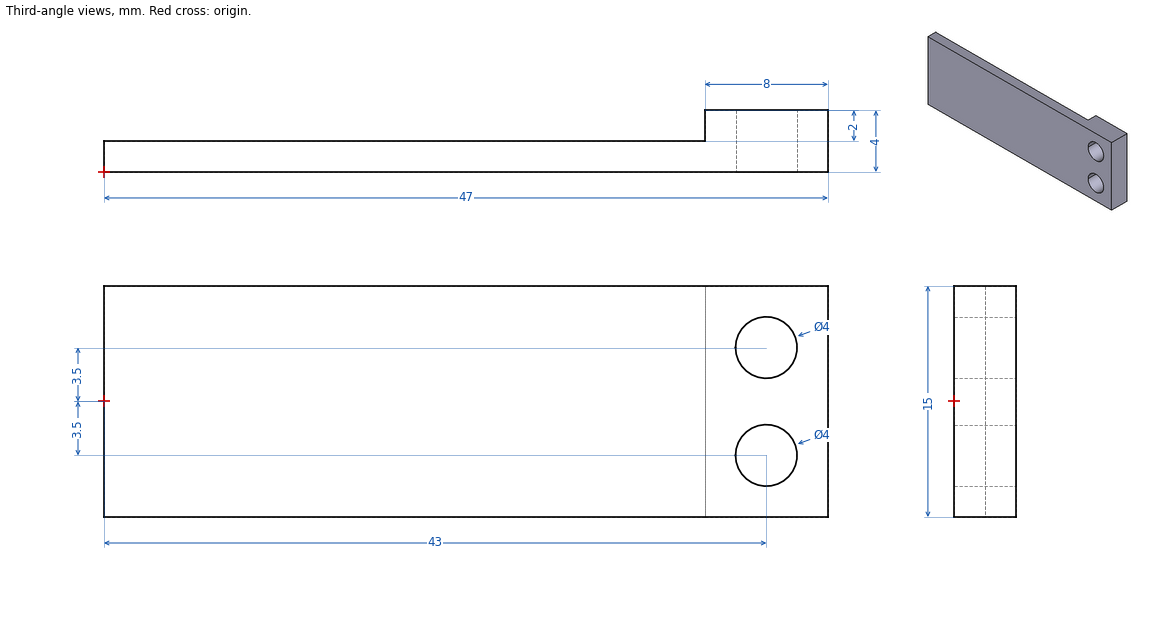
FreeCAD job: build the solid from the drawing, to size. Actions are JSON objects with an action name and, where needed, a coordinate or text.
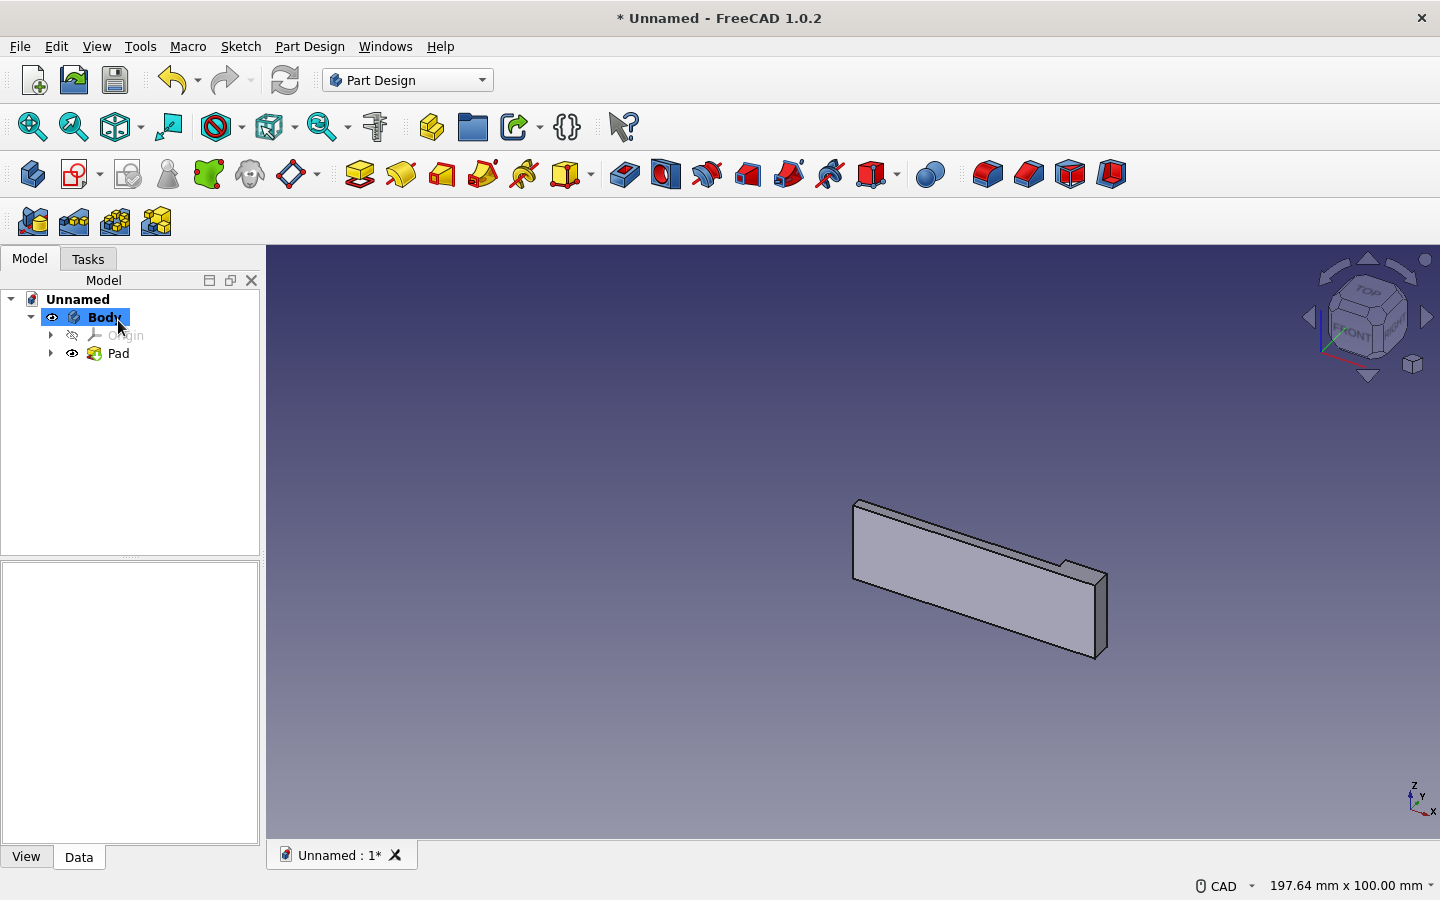
{"action": "left_click", "coordinate": [33, 128]}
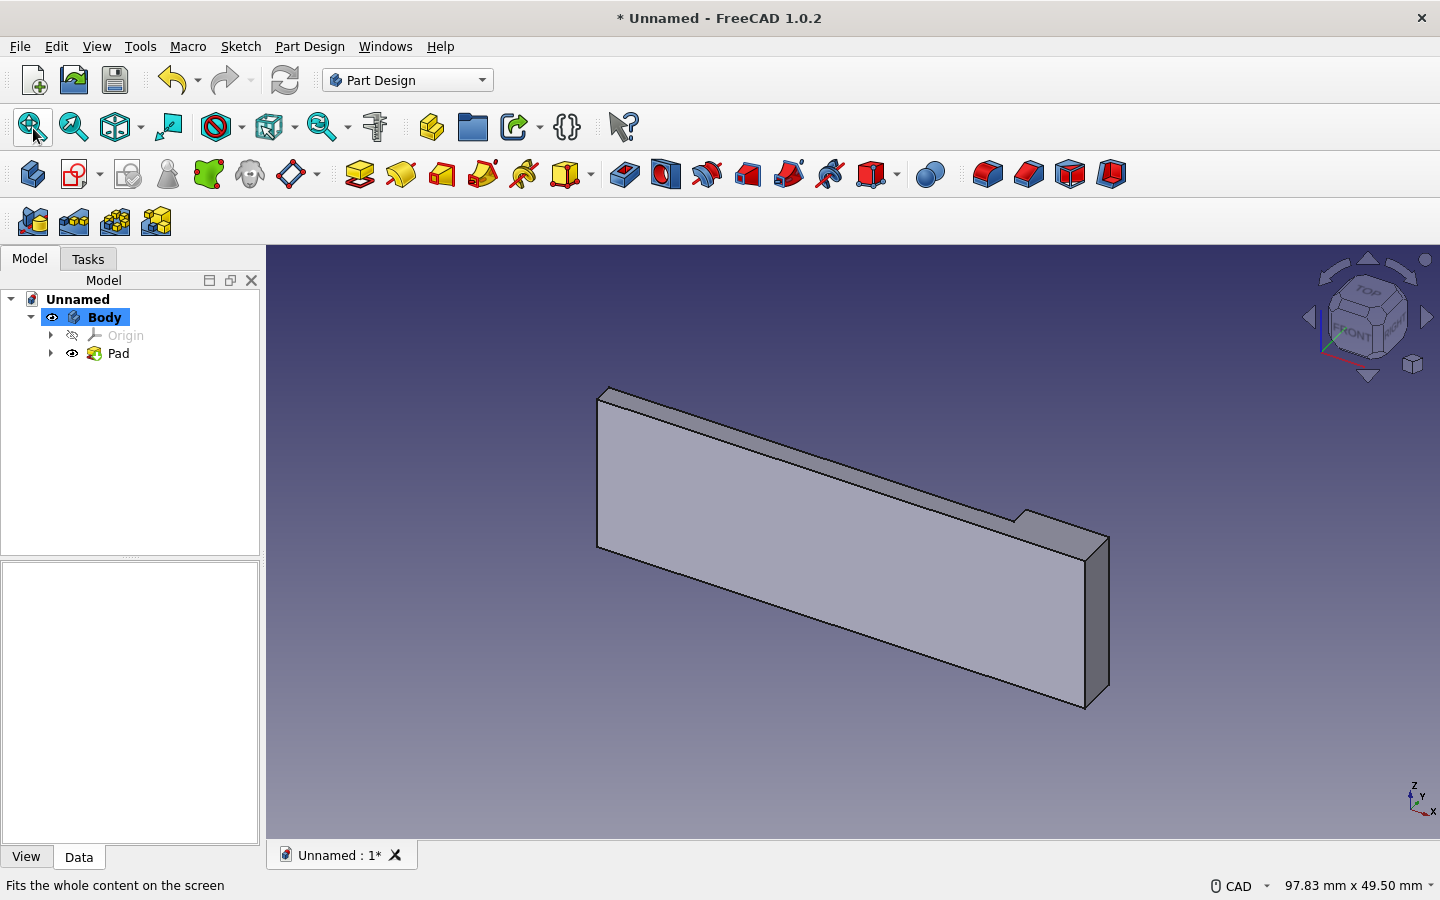
{"action": "key", "text": "4"}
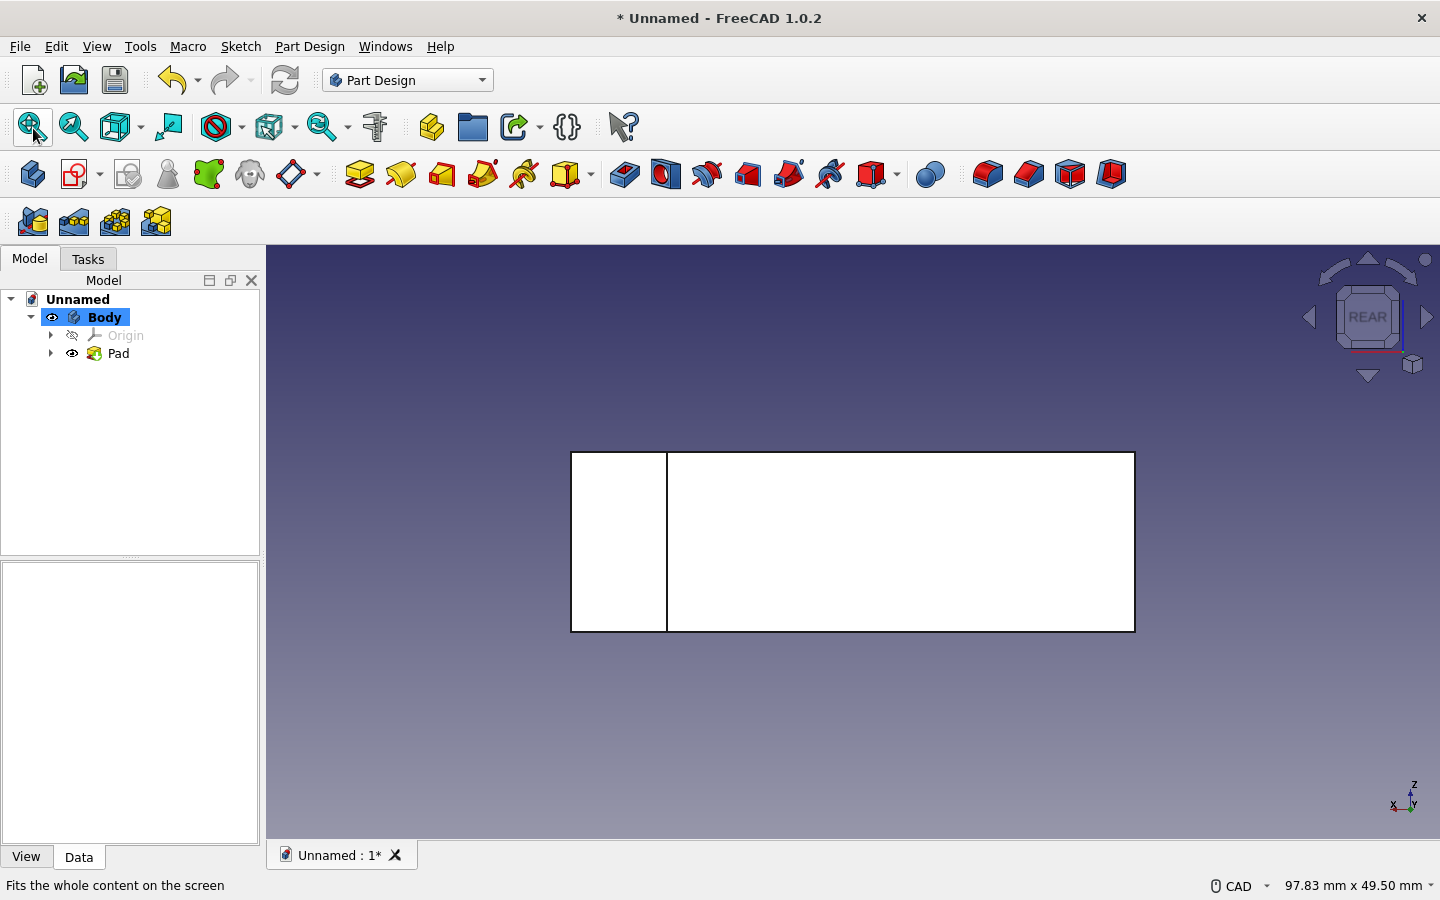
{"action": "left_click", "coordinate": [619, 515]}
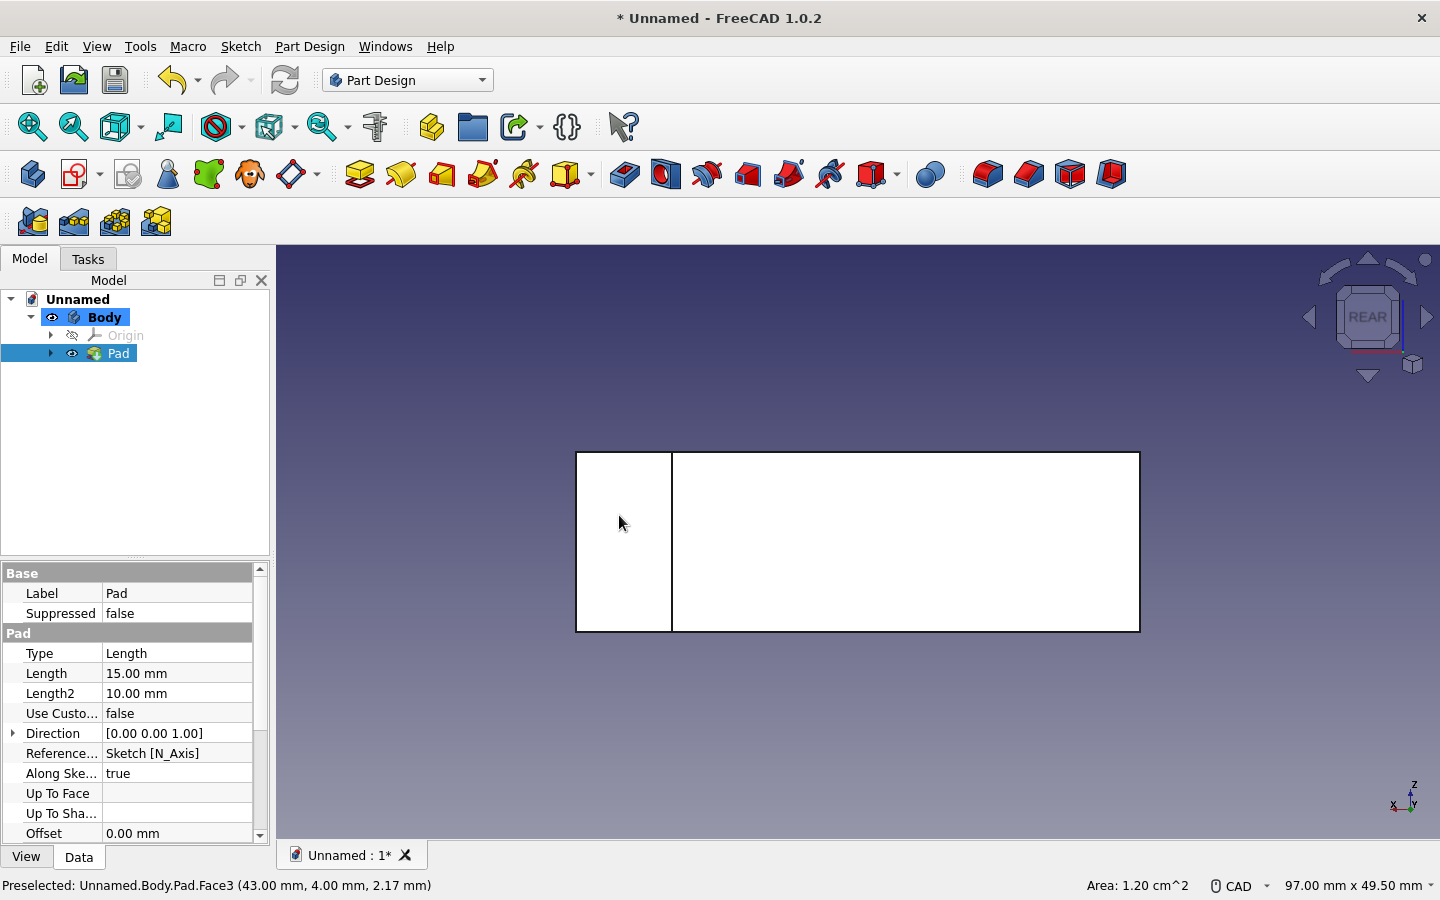
{"action": "left_click", "coordinate": [74, 174]}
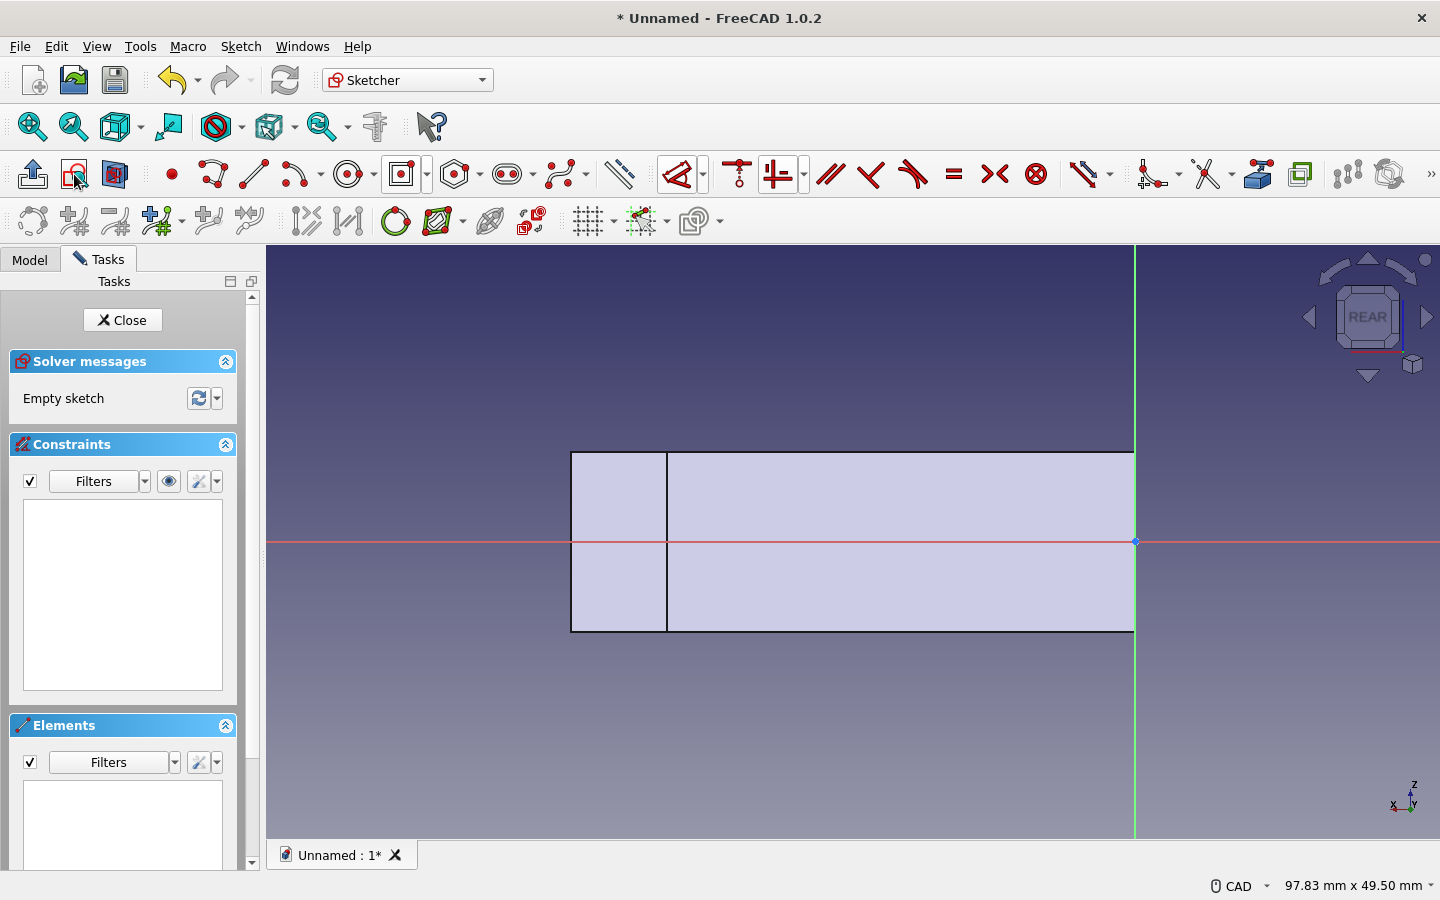
{"action": "scroll", "coordinate": [593, 591], "scroll_direction": "up", "scroll_amount": 10}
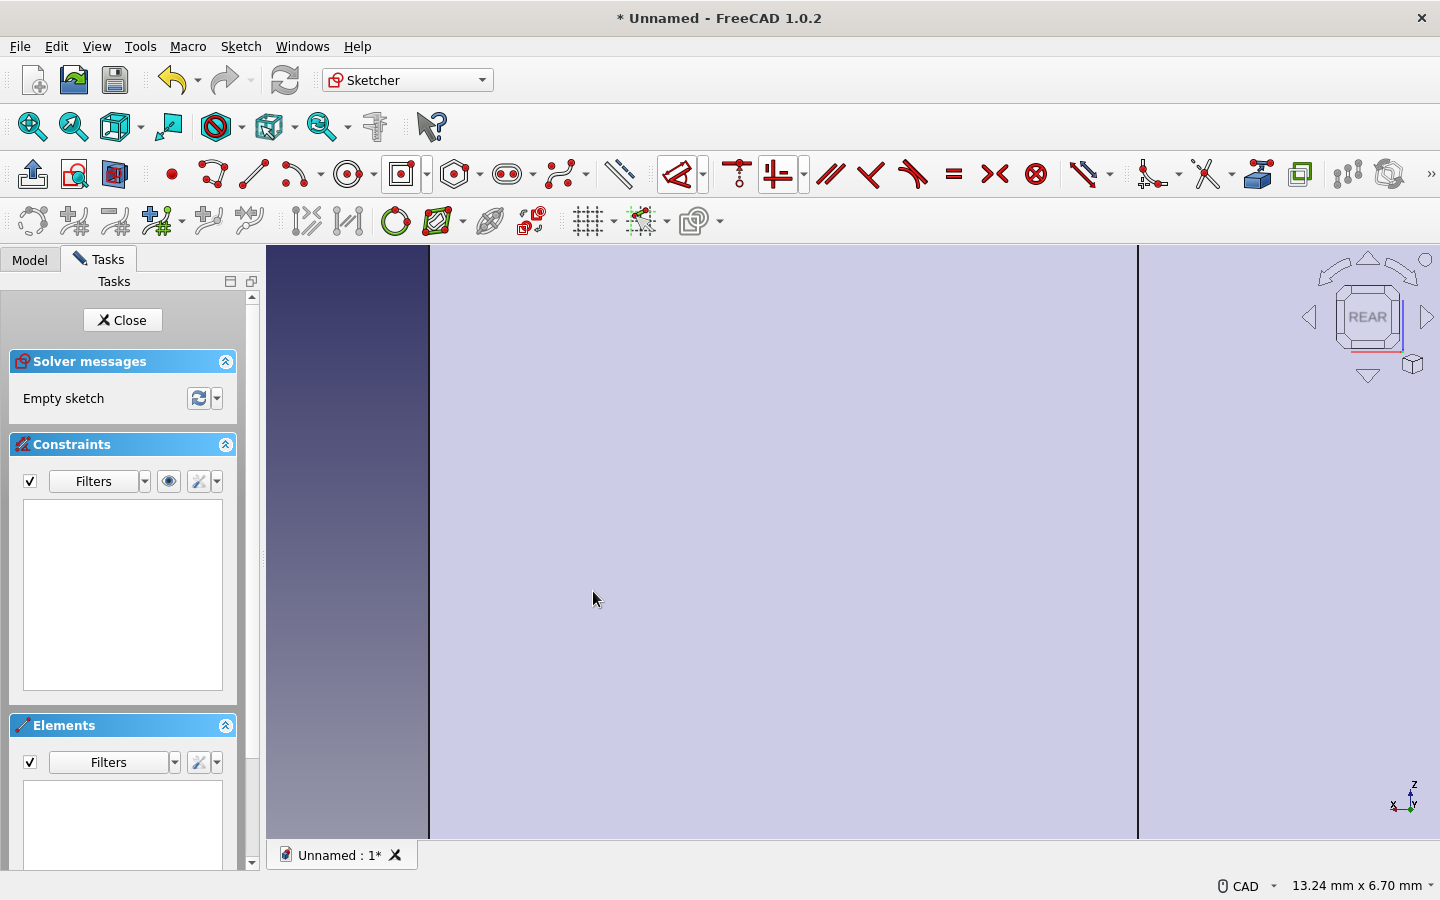
{"action": "left_click", "coordinate": [348, 174]}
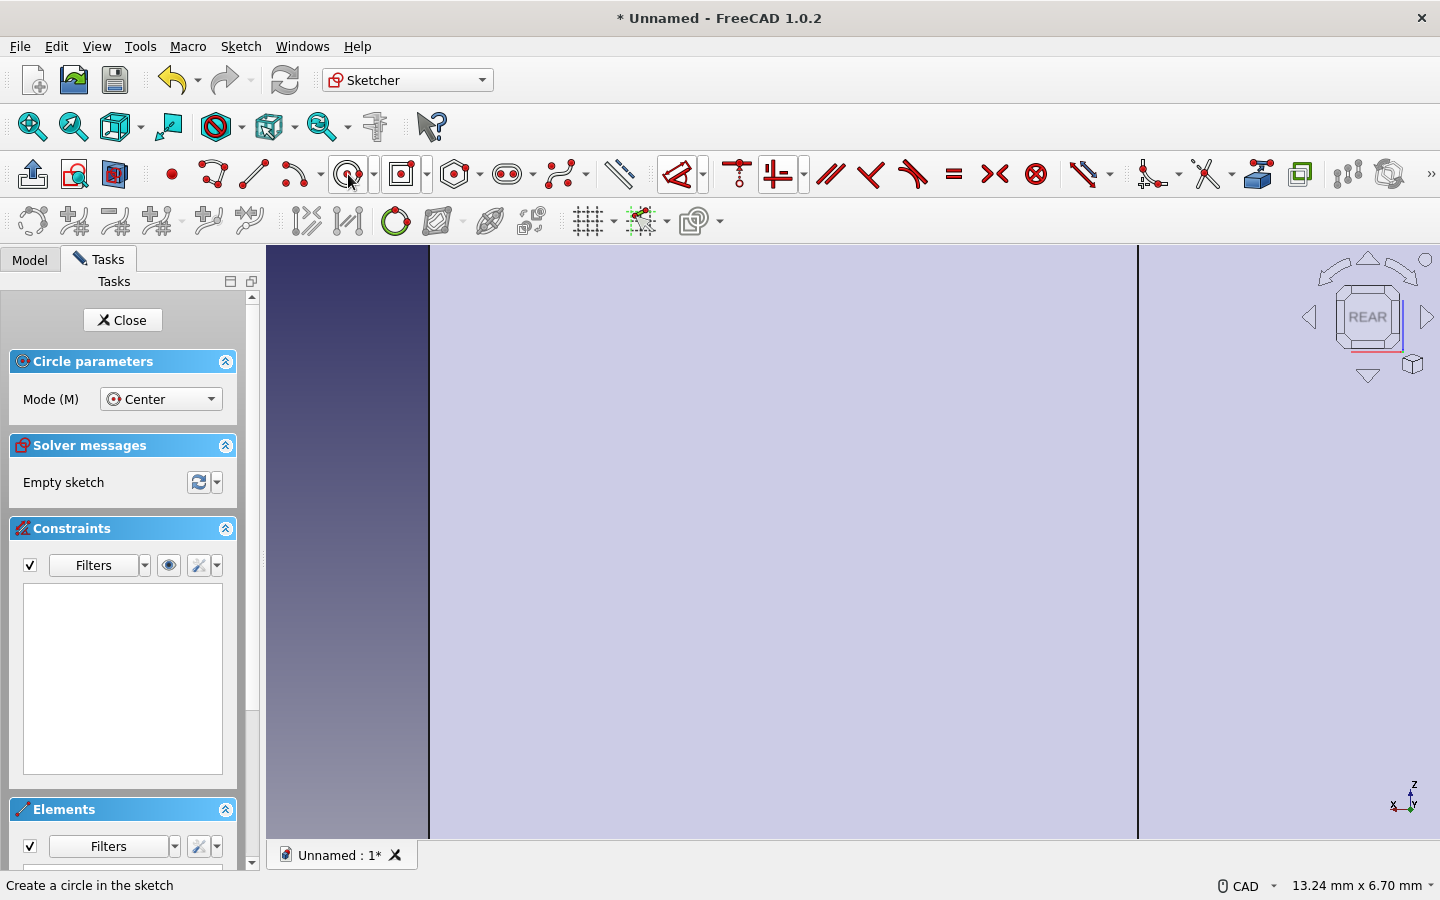
{"action": "left_click", "coordinate": [783, 536]}
{"action": "left_click", "coordinate": [909, 410]}
{"action": "key", "text": "Escape"}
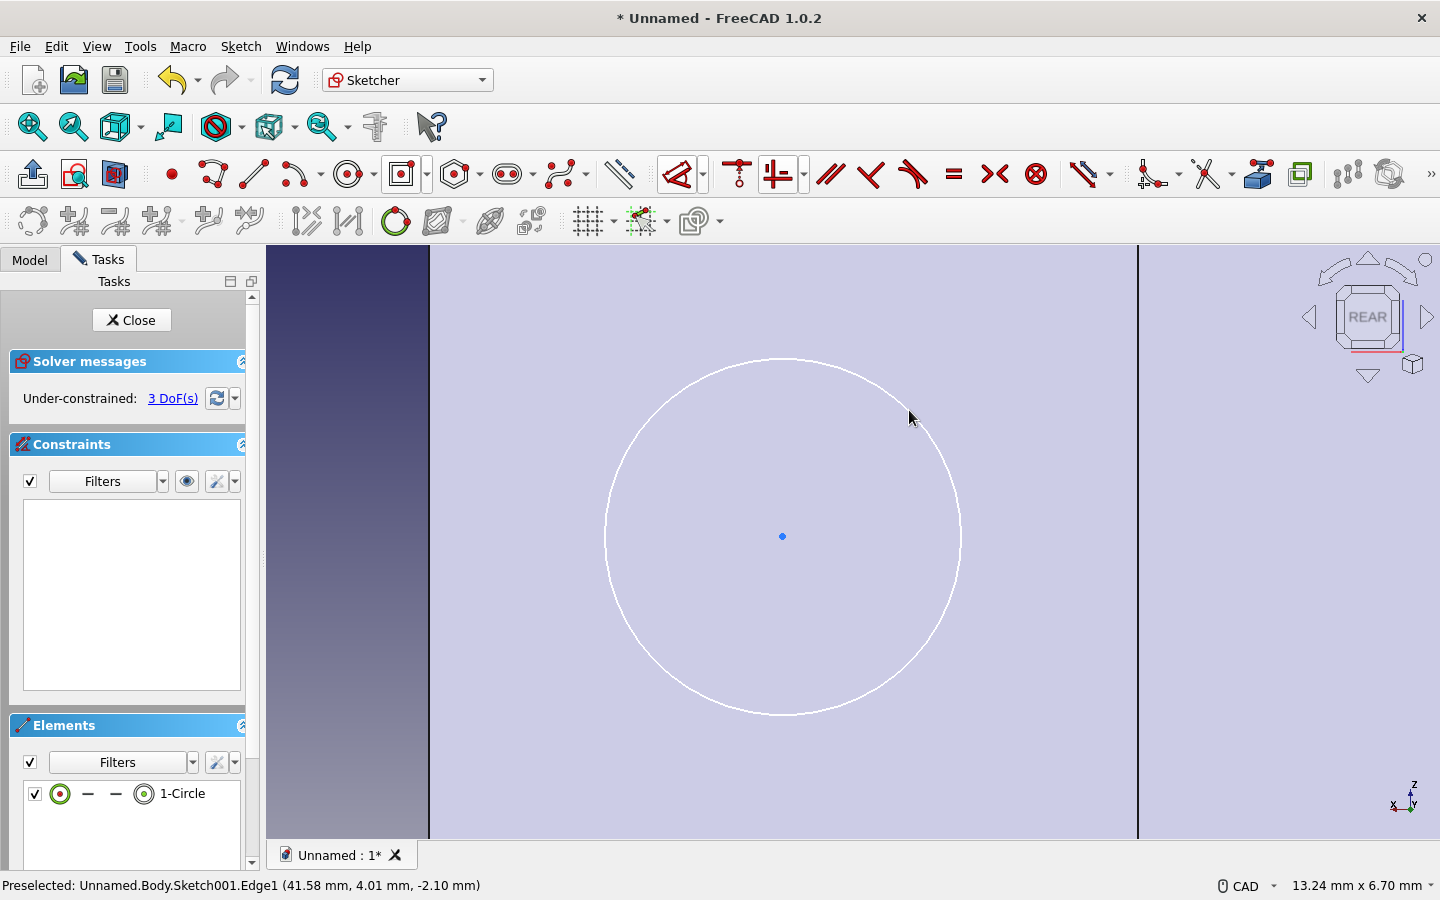
{"action": "left_click", "coordinate": [909, 411]}